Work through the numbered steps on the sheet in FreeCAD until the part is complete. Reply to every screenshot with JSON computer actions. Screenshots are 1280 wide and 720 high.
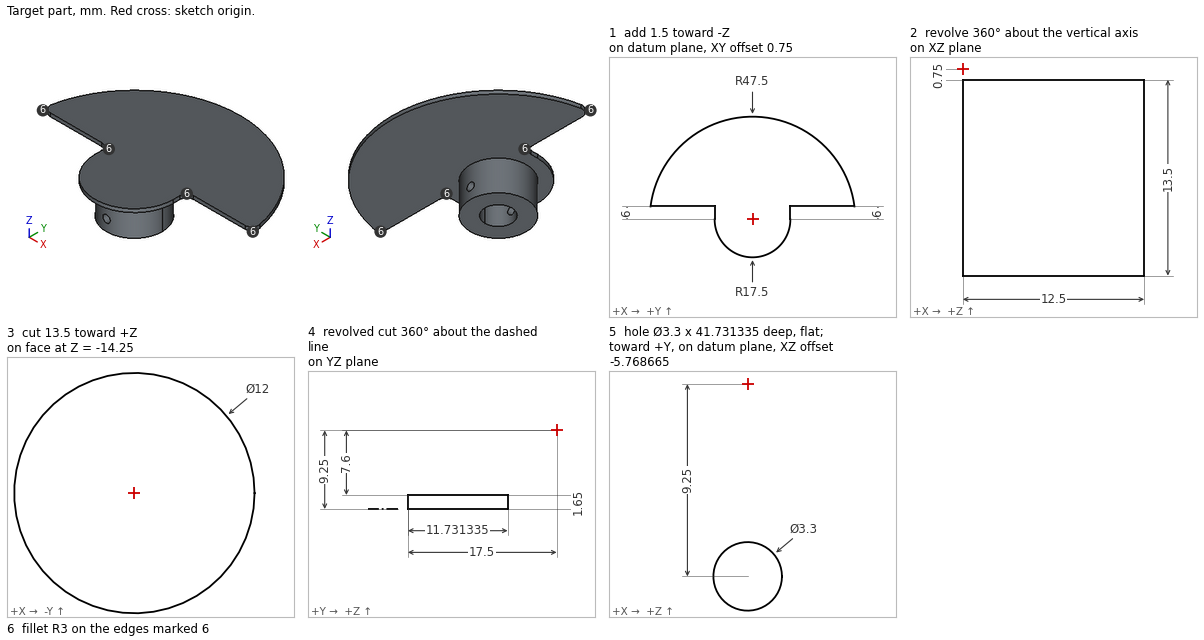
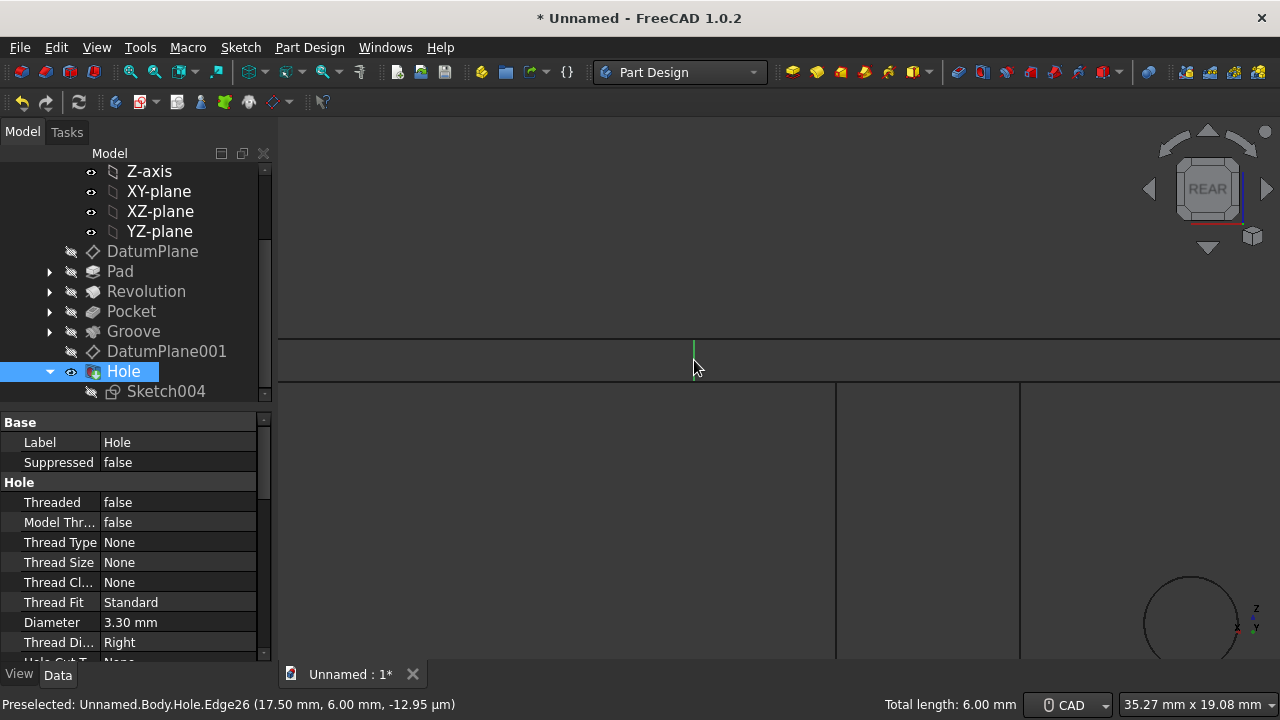
{"action": "key", "text": "v 1"}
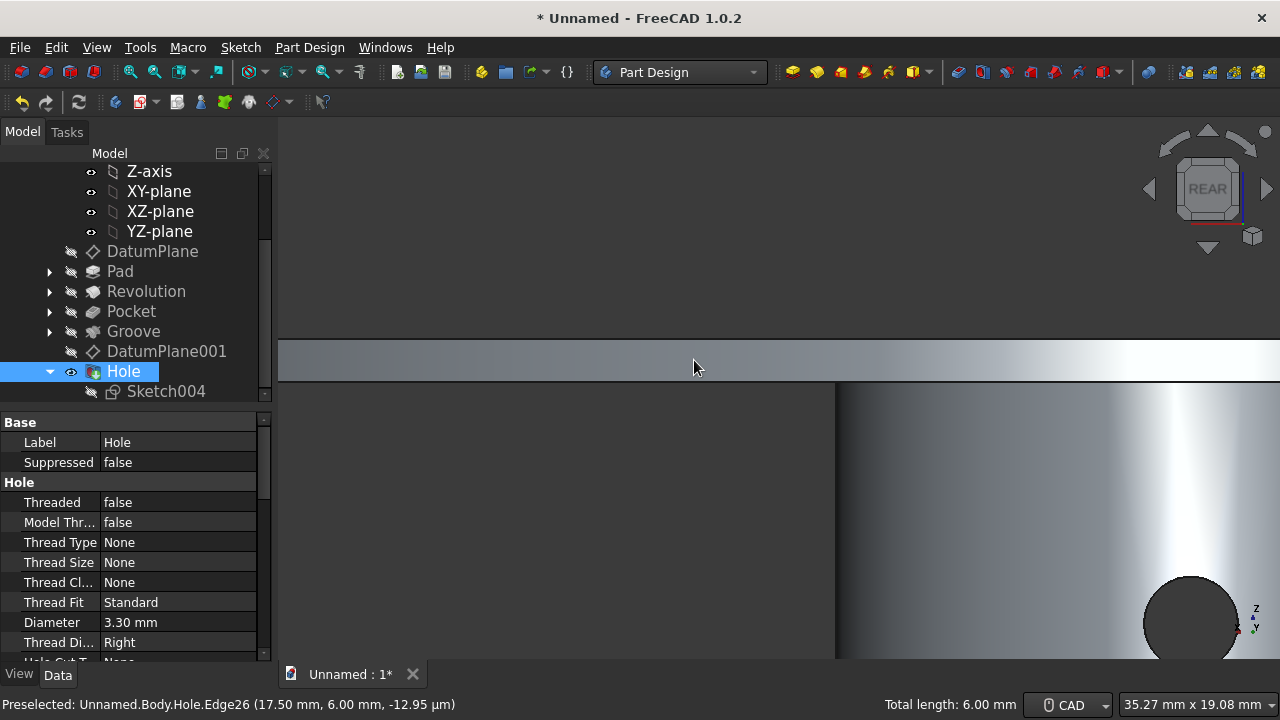
{"action": "left_click", "coordinate": [22, 72]}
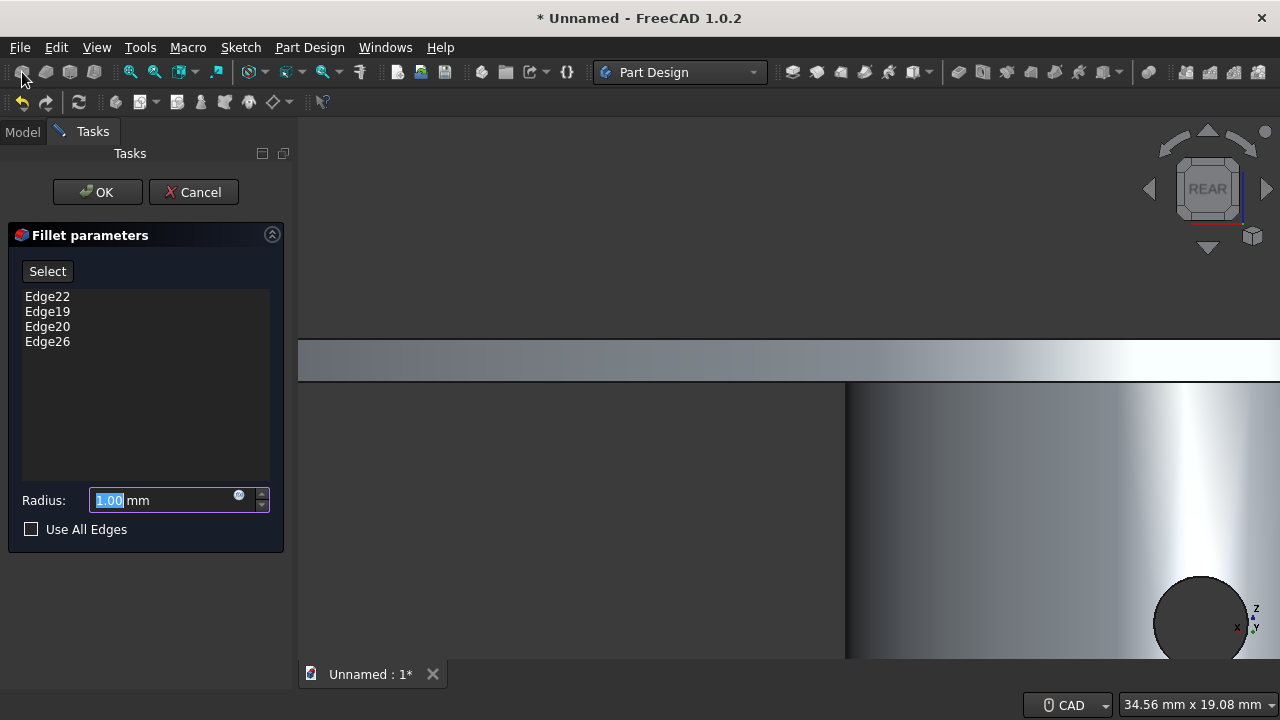
{"action": "type", "text": "3"}
{"action": "key", "text": "Tab"}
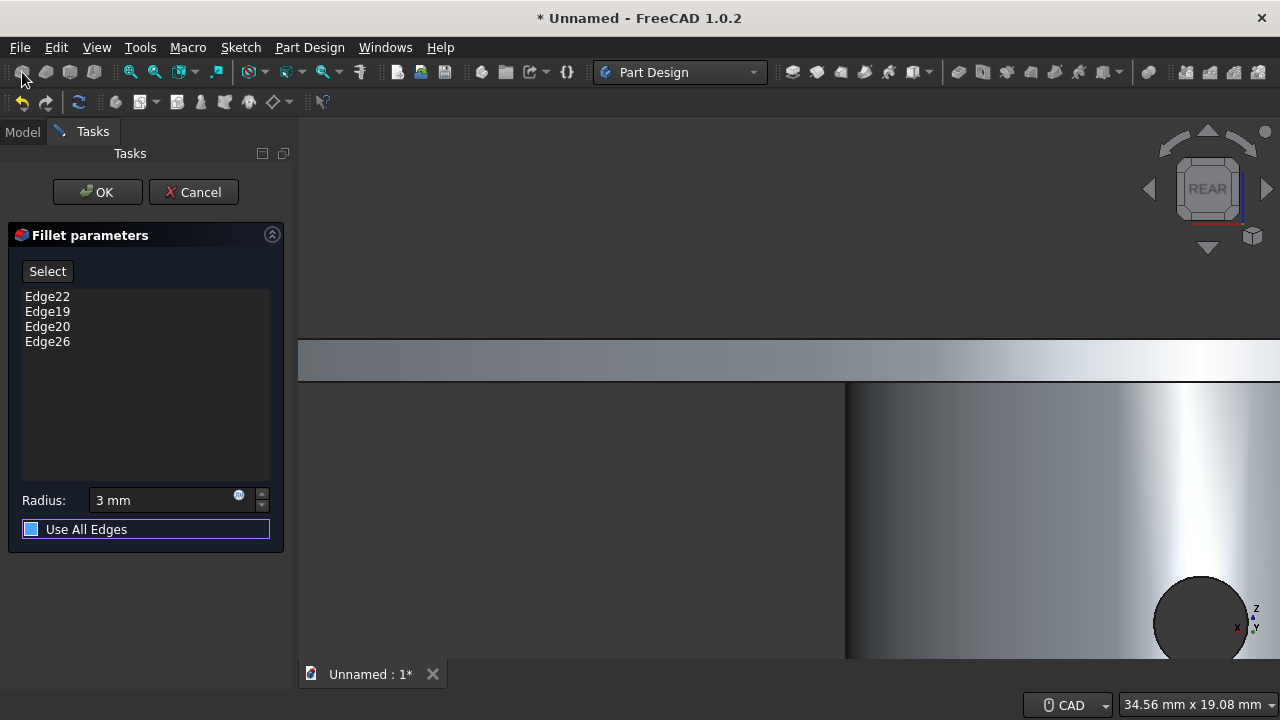
{"action": "left_click", "coordinate": [98, 192]}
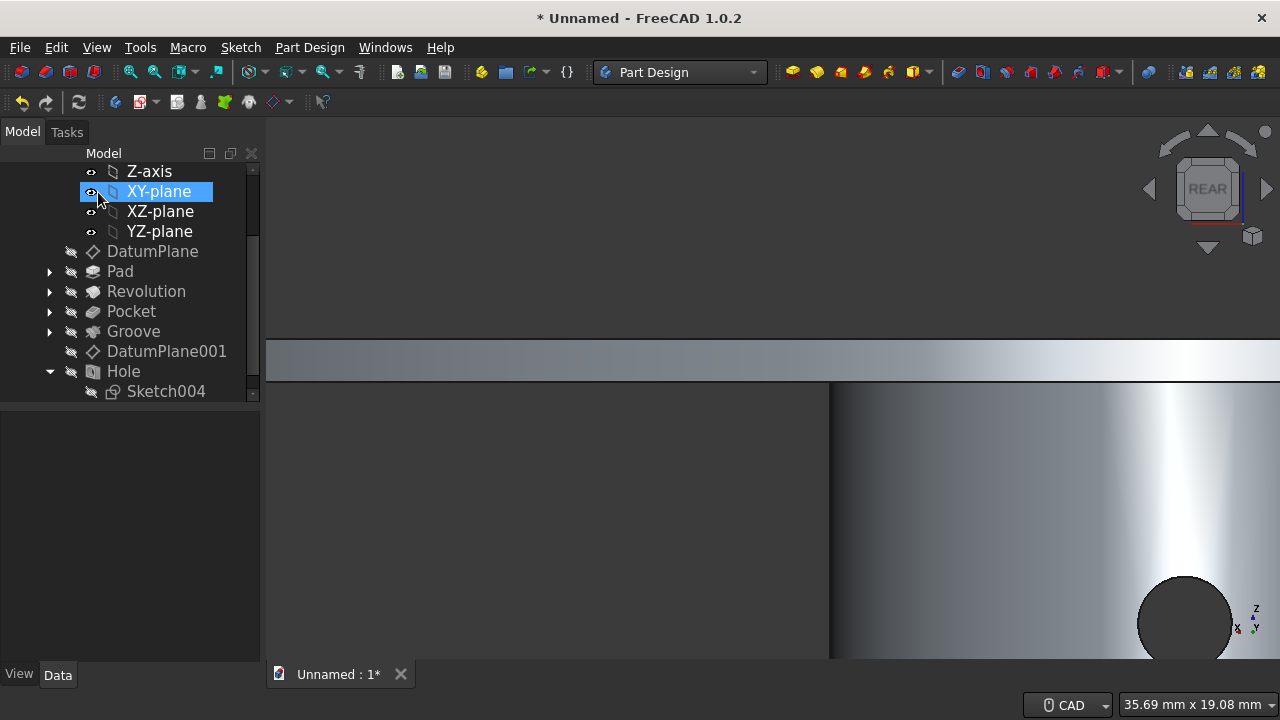
{"action": "key", "text": "0"}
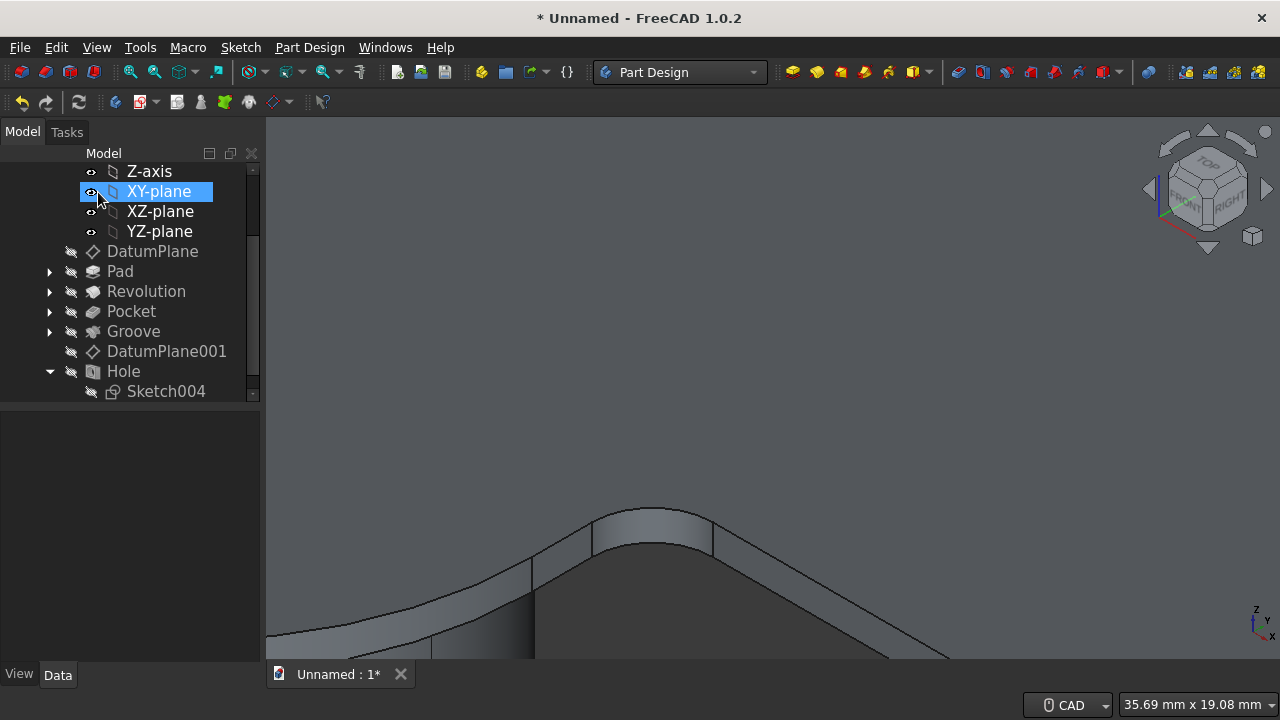
{"action": "key", "text": "v f"}